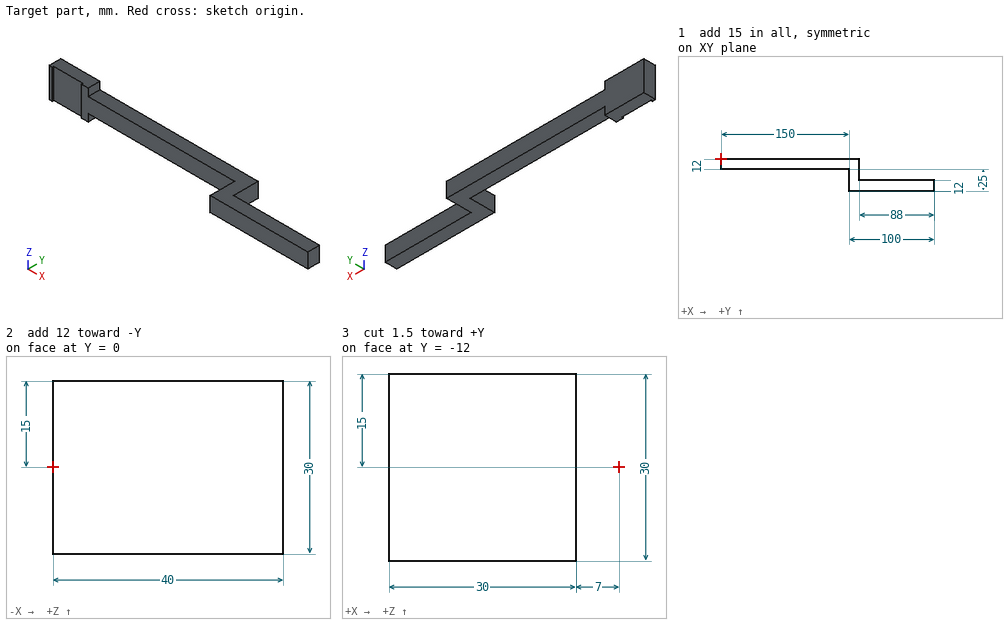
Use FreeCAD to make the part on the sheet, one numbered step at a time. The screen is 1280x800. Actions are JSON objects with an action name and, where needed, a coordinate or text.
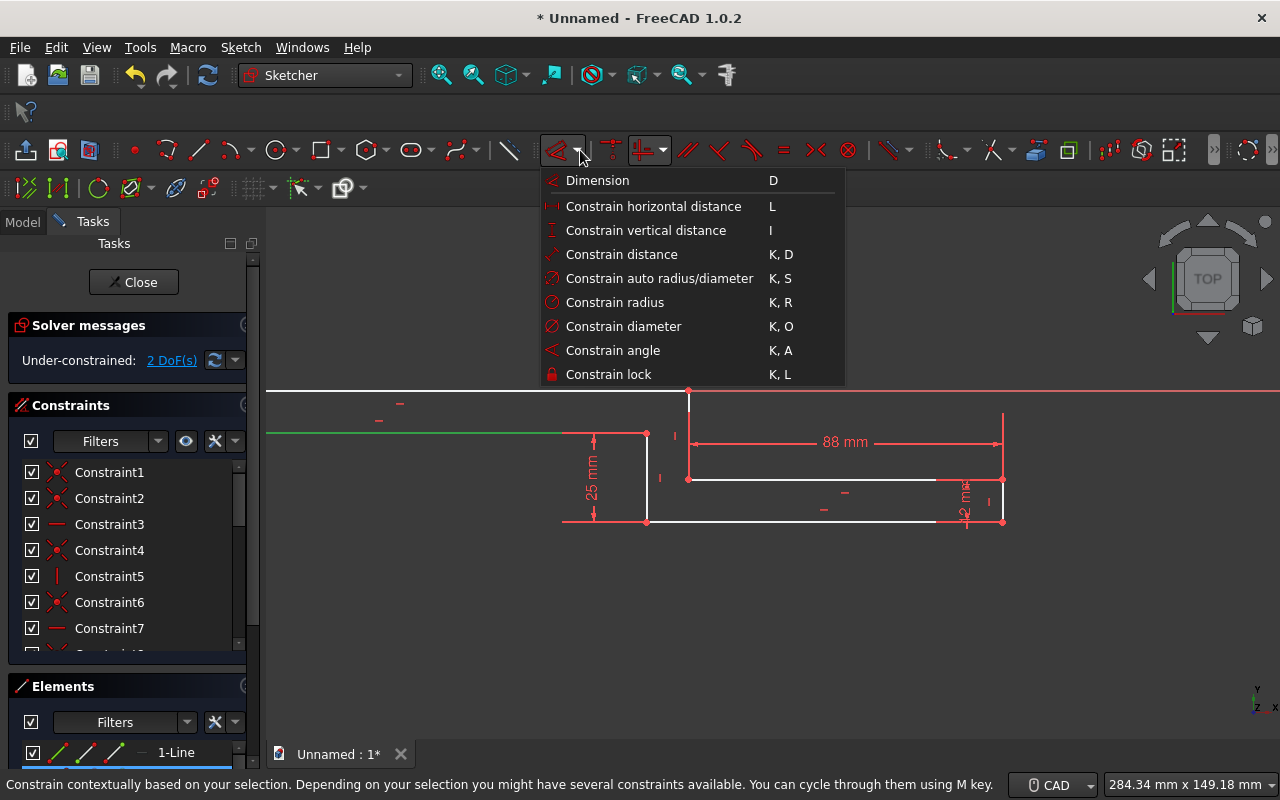
{"action": "left_click", "coordinate": [693, 206]}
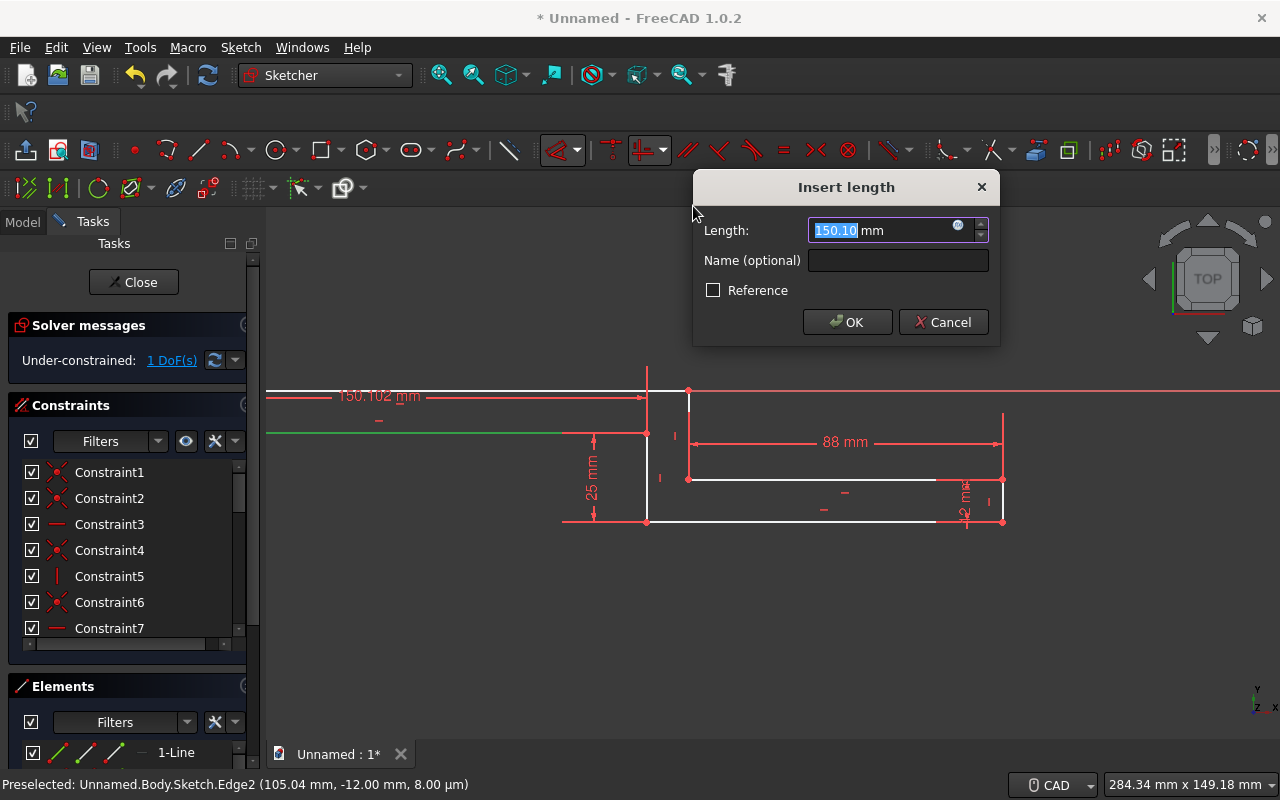
{"action": "type", "text": "150"}
{"action": "key", "text": "Return"}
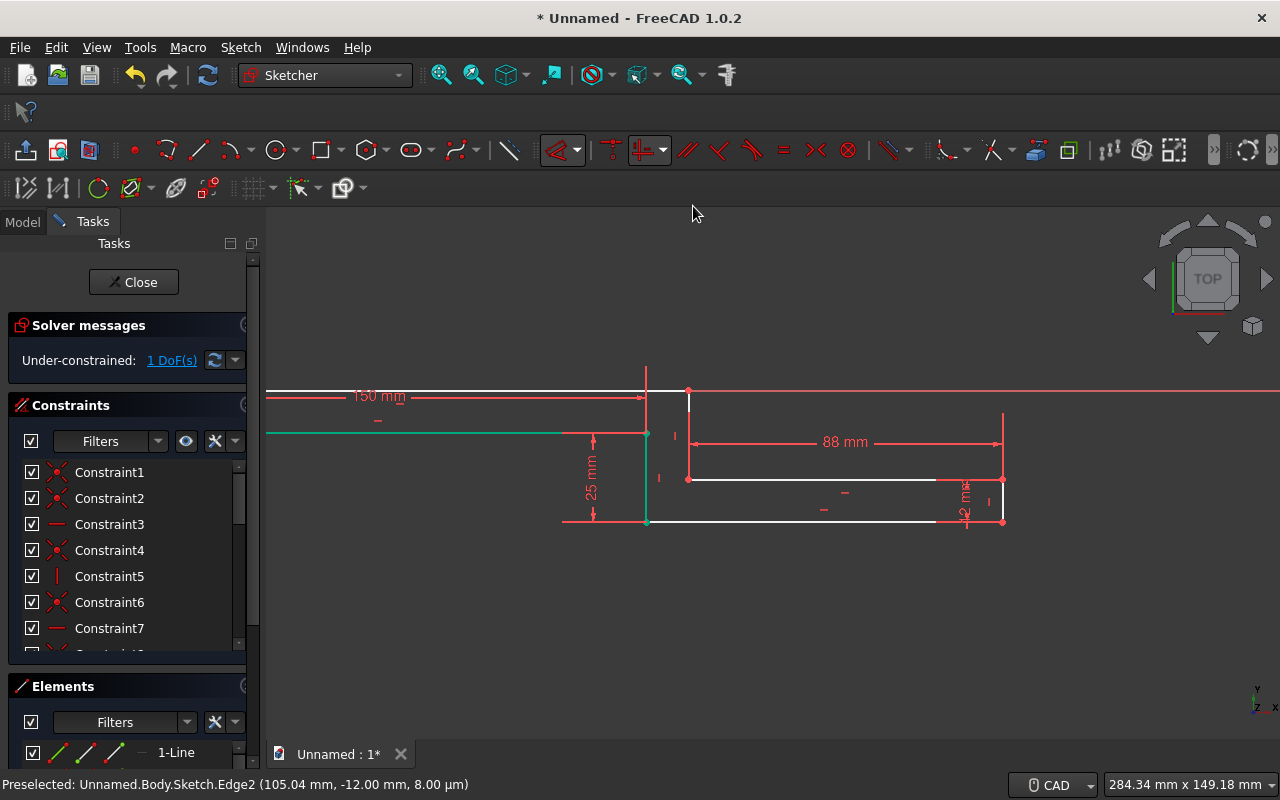
{"action": "left_click", "coordinate": [753, 522]}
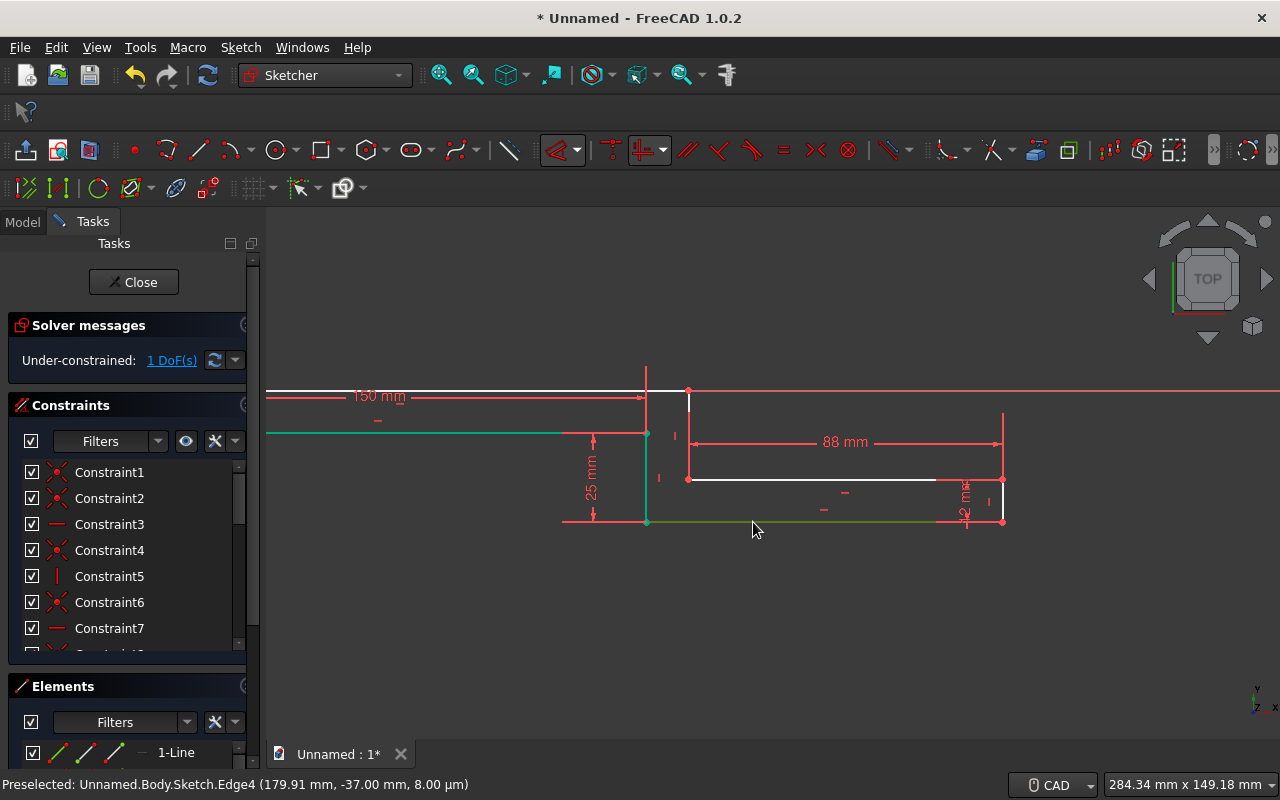
{"action": "left_click", "coordinate": [580, 150]}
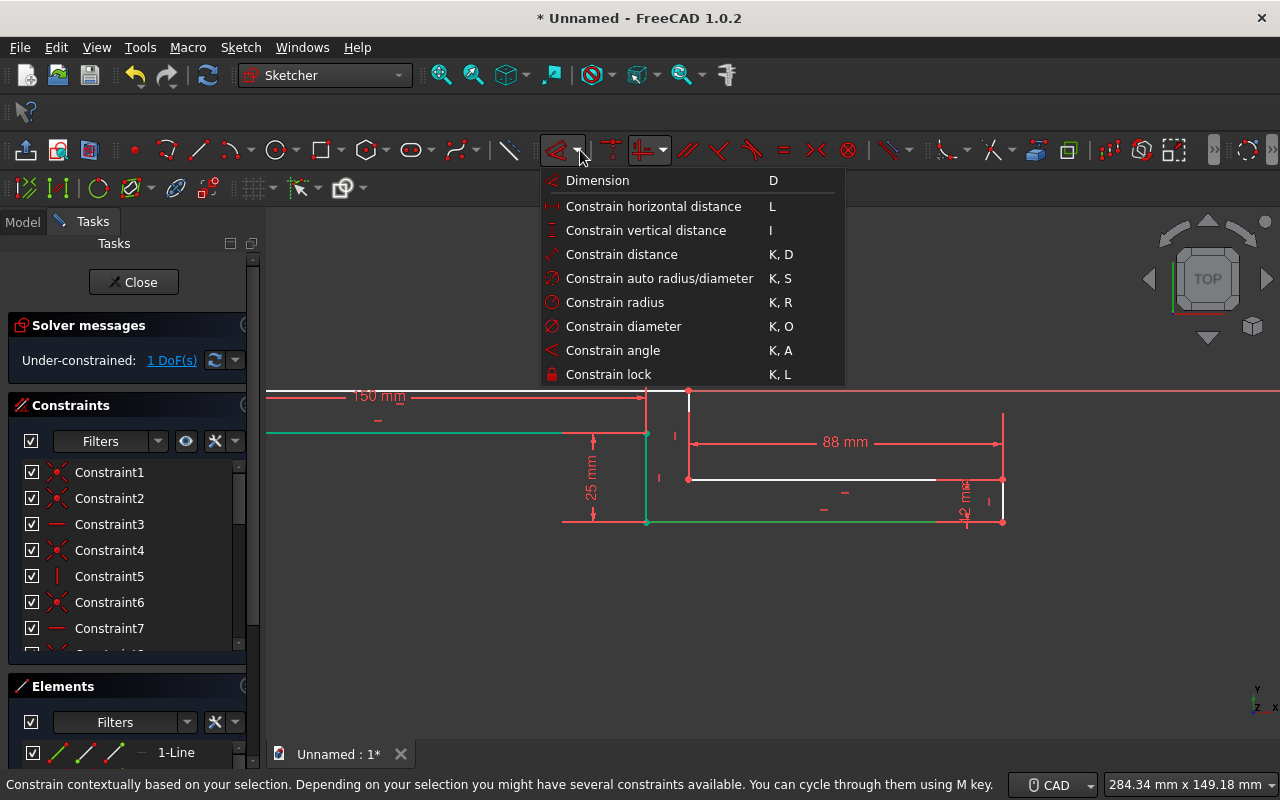
{"action": "left_click", "coordinate": [693, 206]}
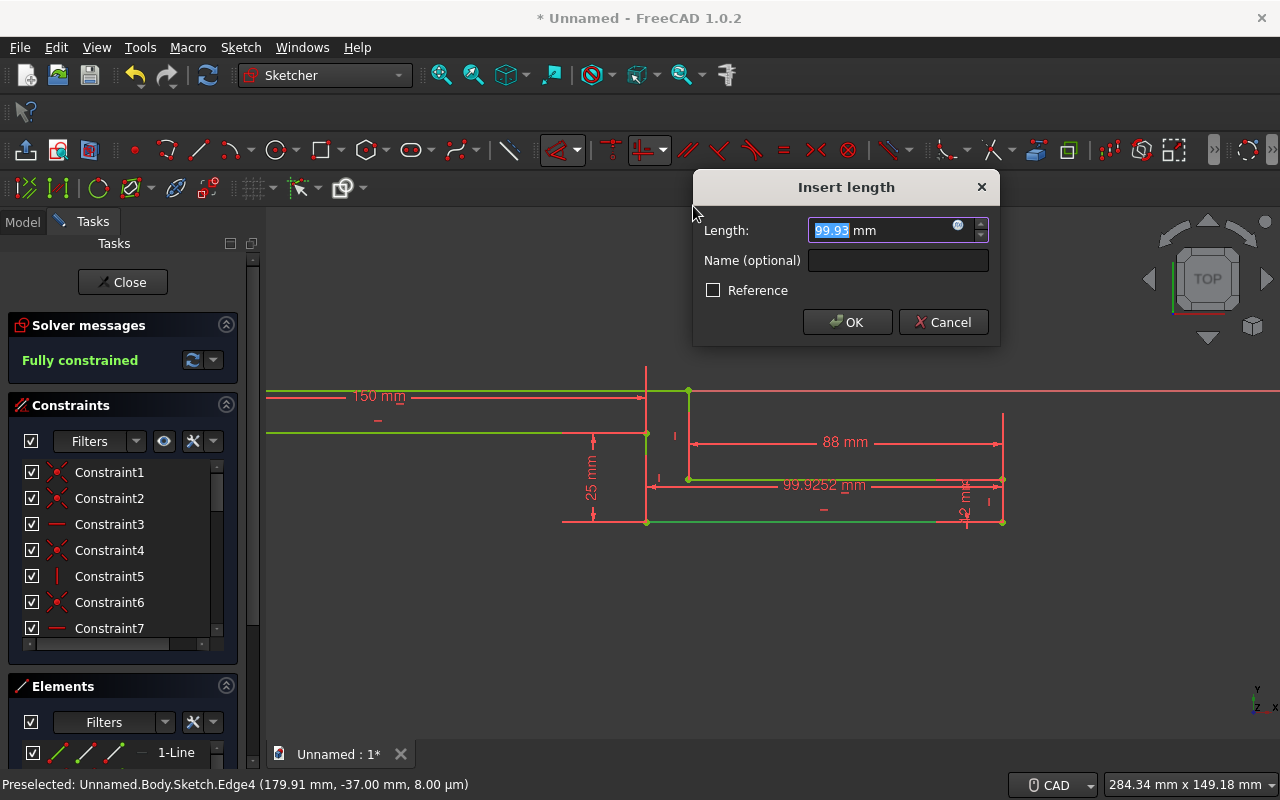
{"action": "type", "text": "100"}
{"action": "key", "text": "Return"}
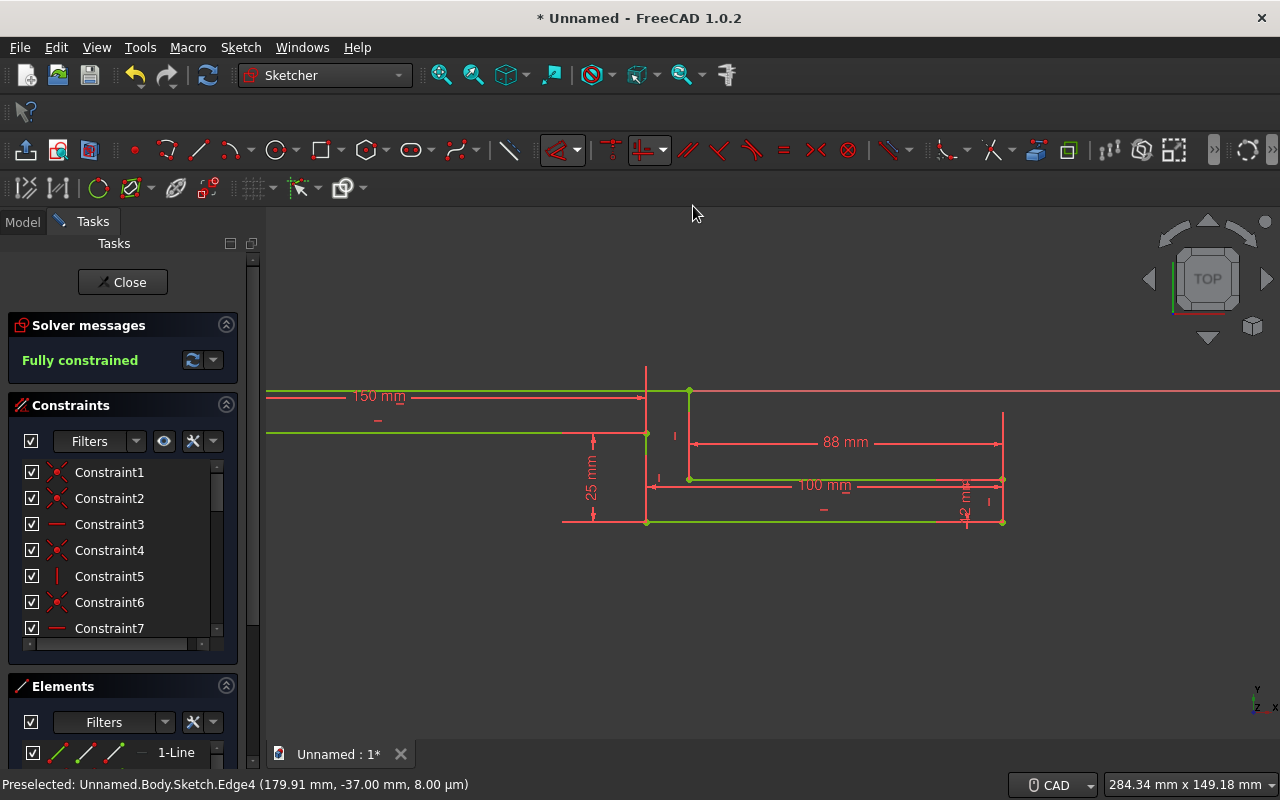
{"action": "left_click", "coordinate": [123, 282]}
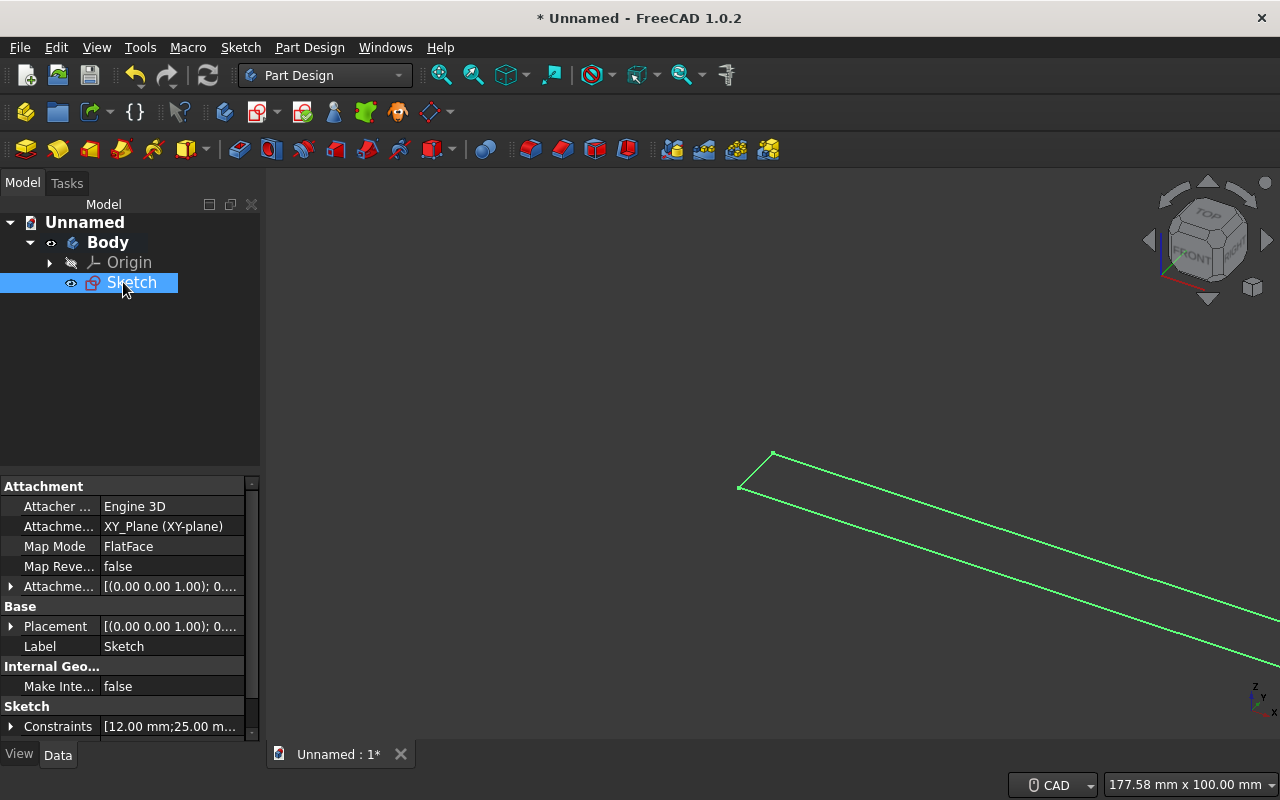
{"action": "left_click", "coordinate": [26, 150]}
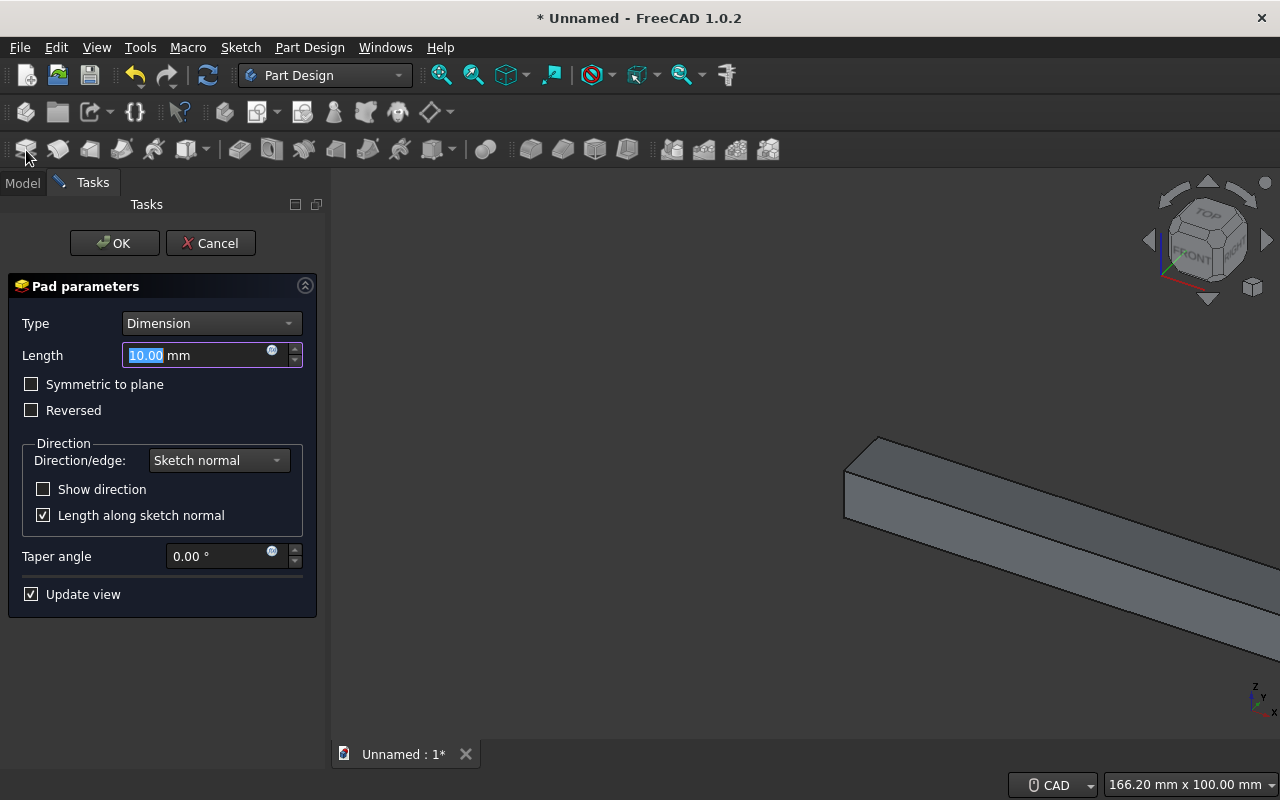
{"action": "type", "text": "15"}
{"action": "key", "text": "Tab"}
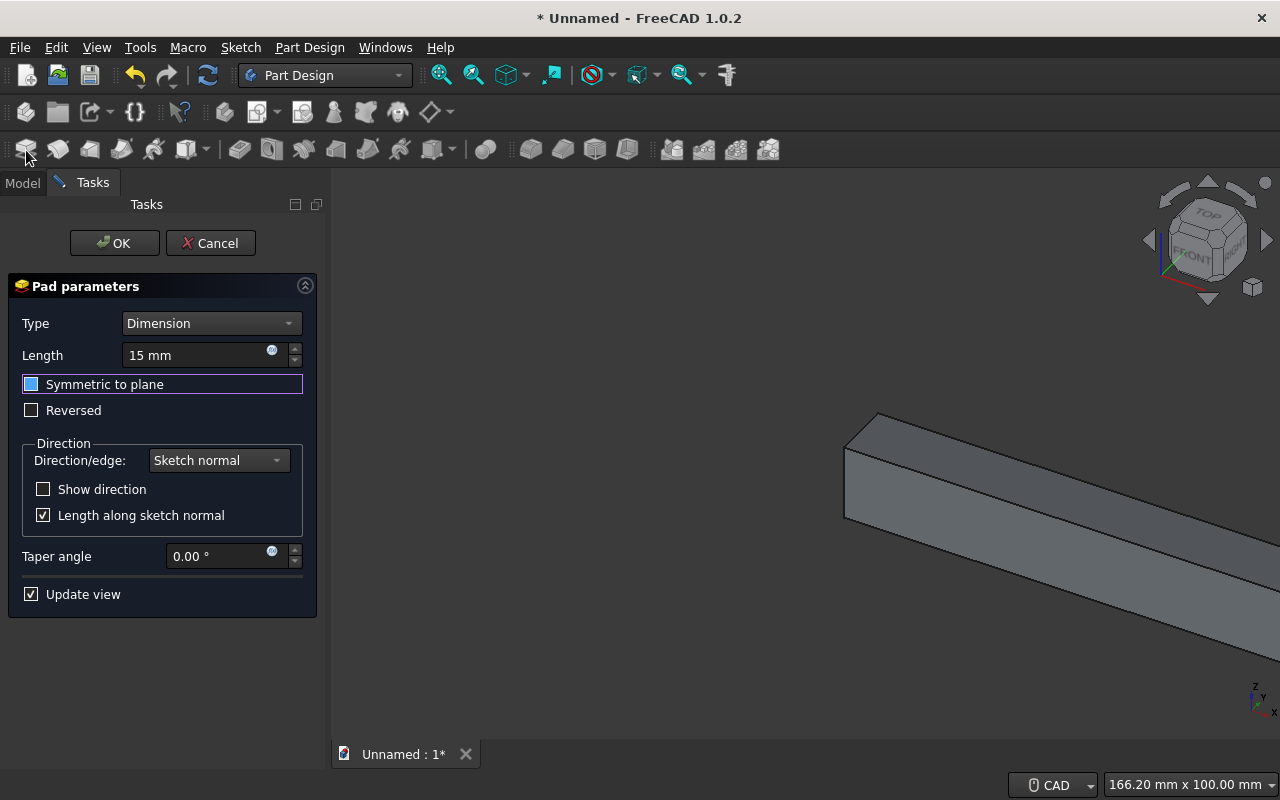
{"action": "left_click", "coordinate": [30, 384]}